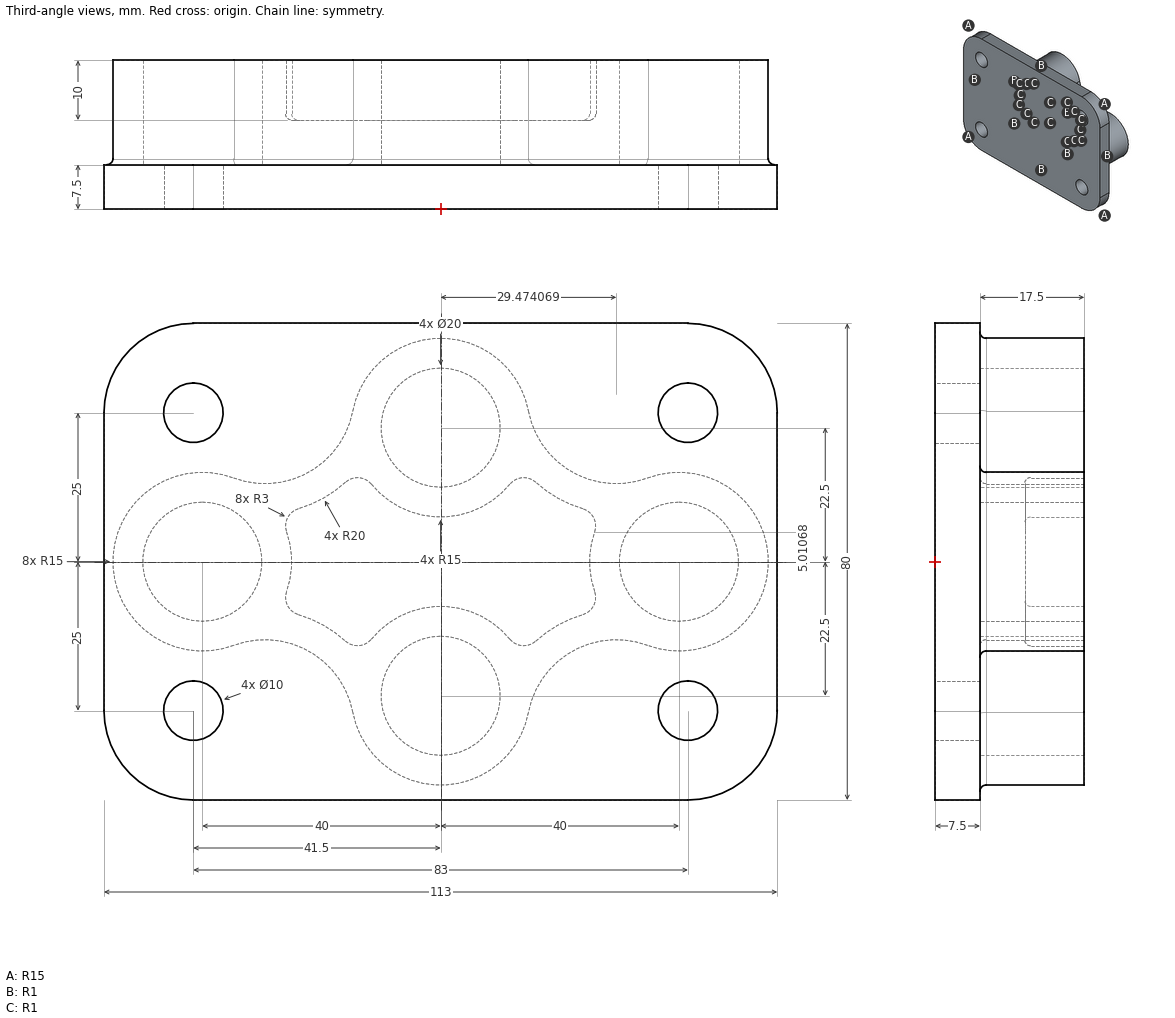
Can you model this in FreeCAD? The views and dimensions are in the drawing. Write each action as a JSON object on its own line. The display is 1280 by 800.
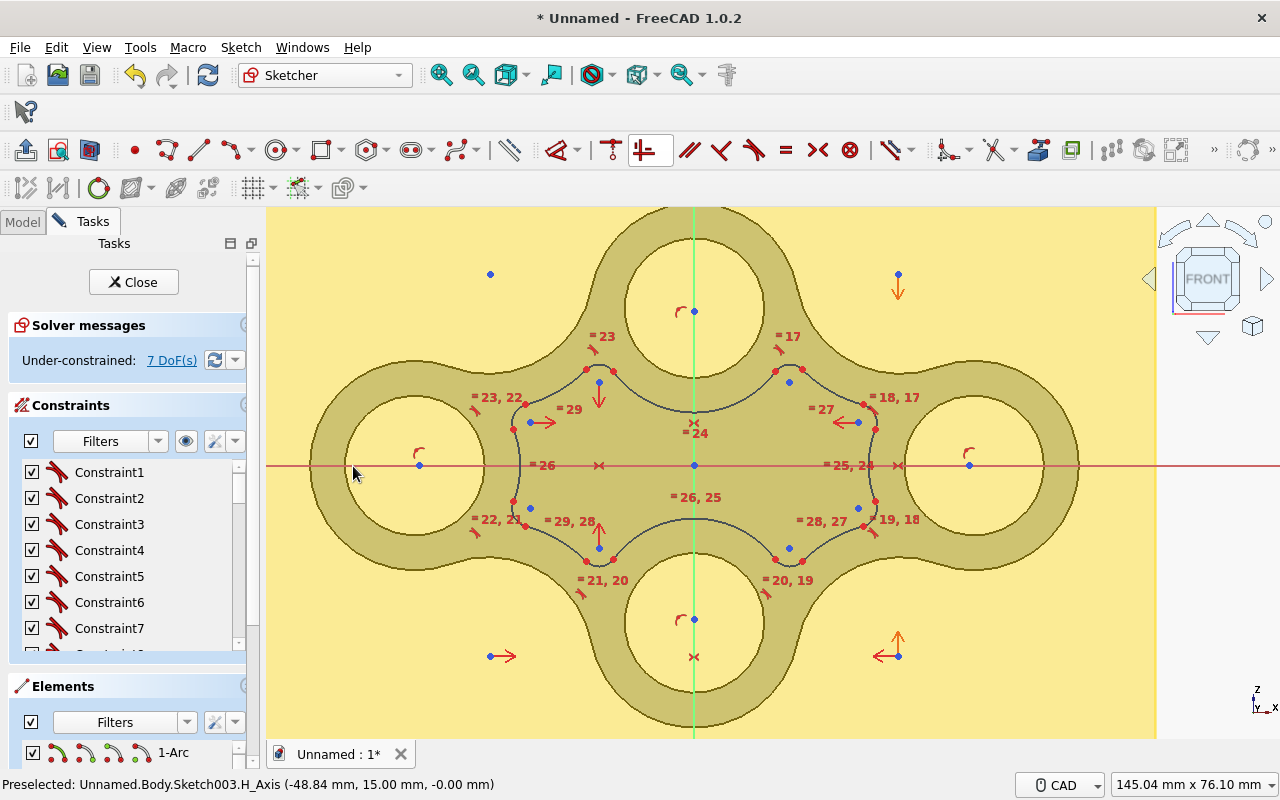
{"action": "left_click", "coordinate": [658, 406]}
{"action": "left_click", "coordinate": [646, 436]}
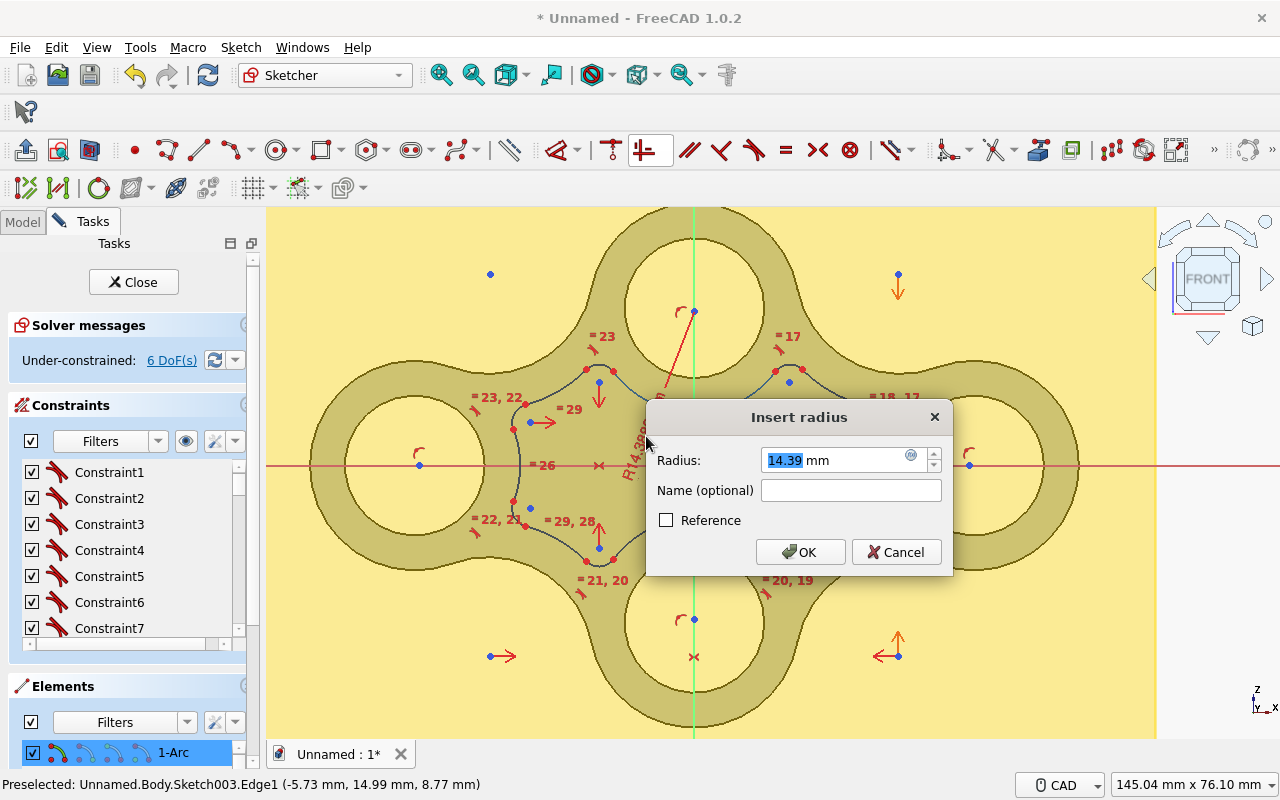
{"action": "type", "text": "15"}
{"action": "key", "text": "Return"}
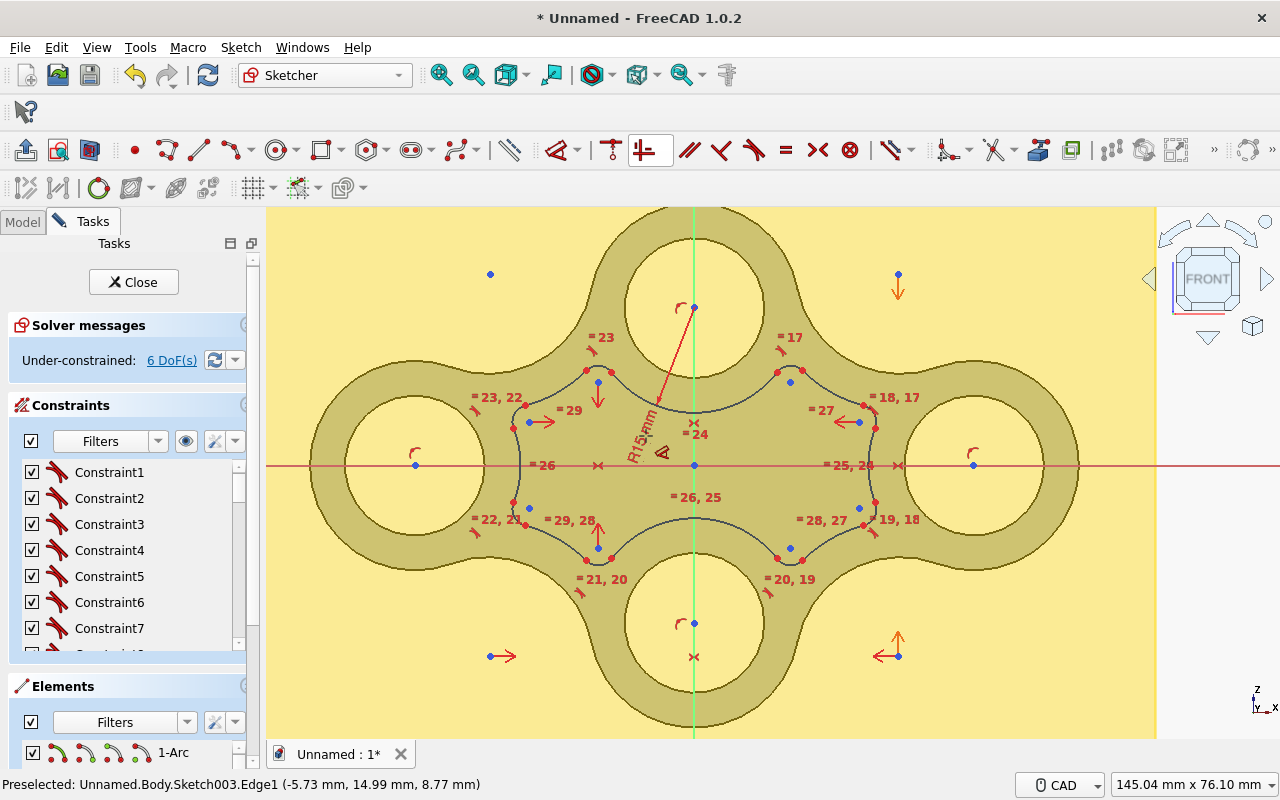
{"action": "scroll", "coordinate": [790, 366], "scroll_direction": "up", "scroll_amount": 4}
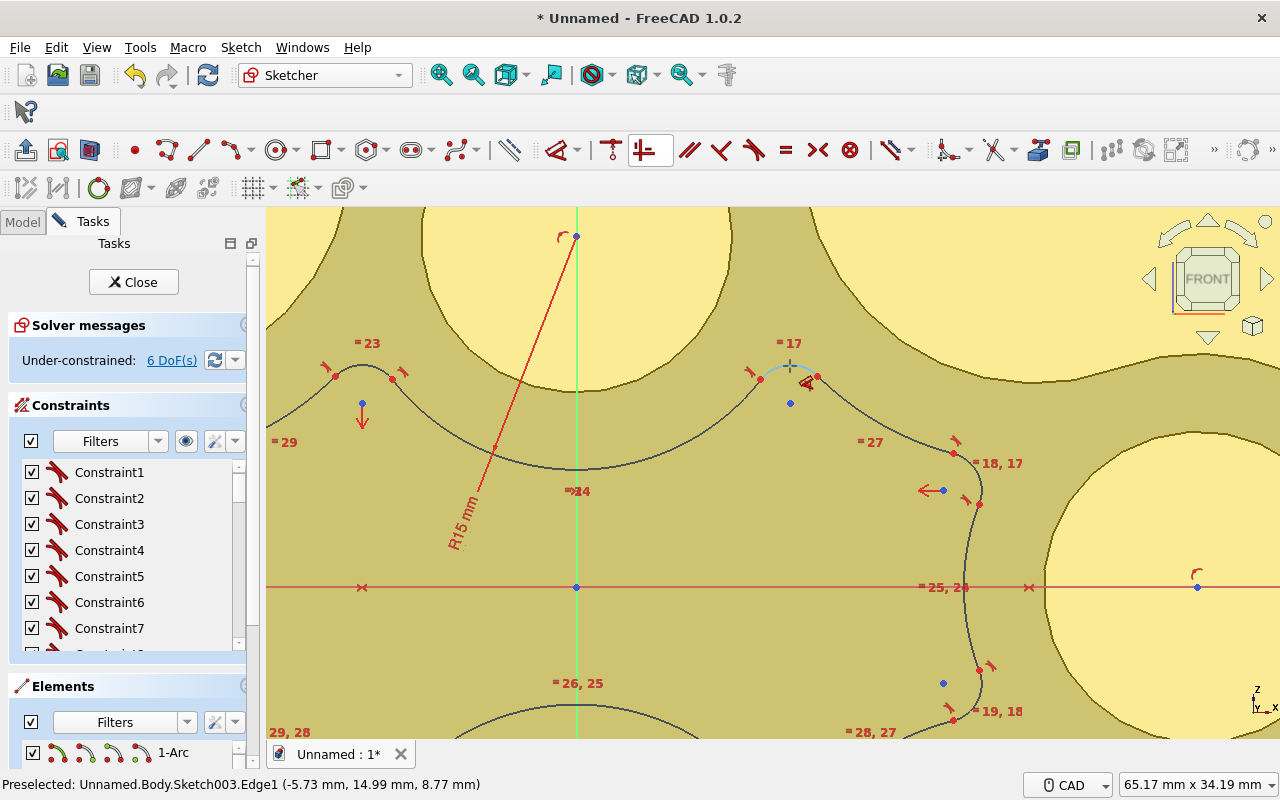
{"action": "left_click", "coordinate": [789, 365]}
{"action": "left_click", "coordinate": [787, 333]}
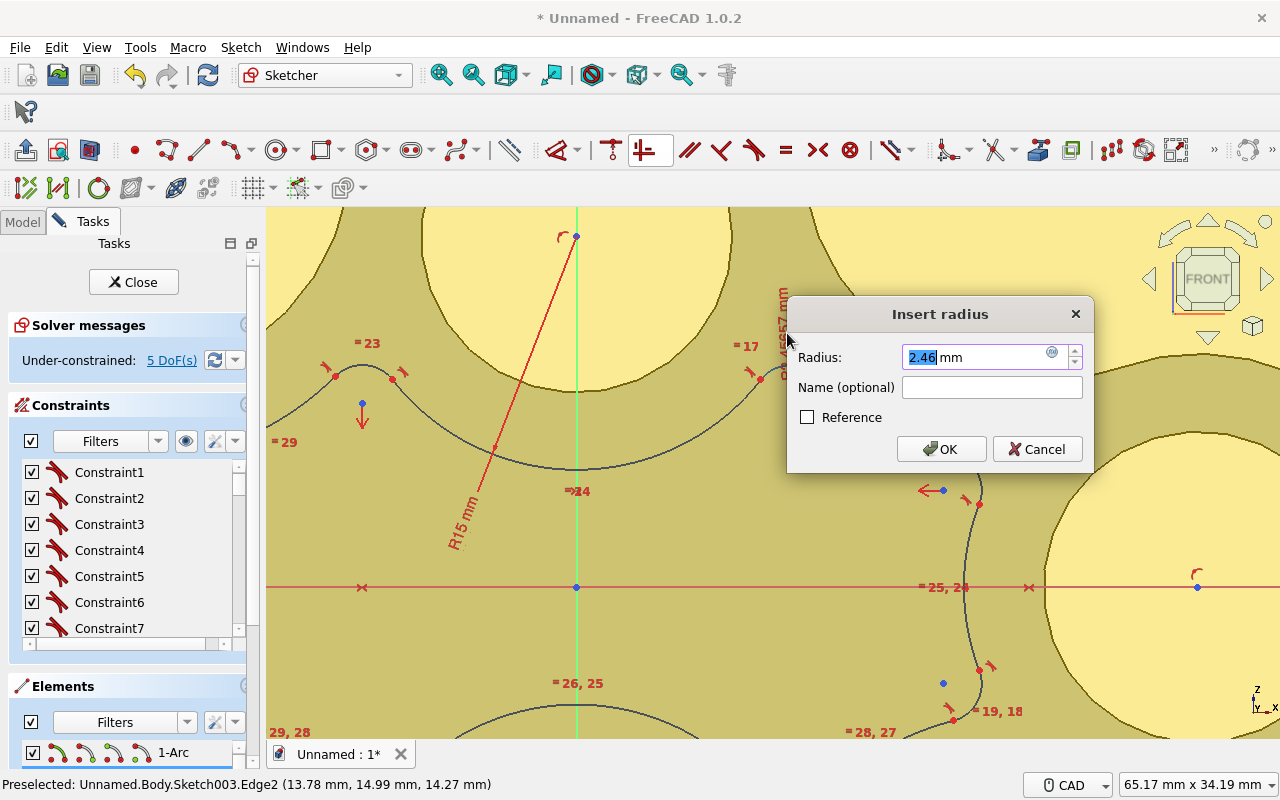
{"action": "type", "text": "3"}
{"action": "key", "text": "Return"}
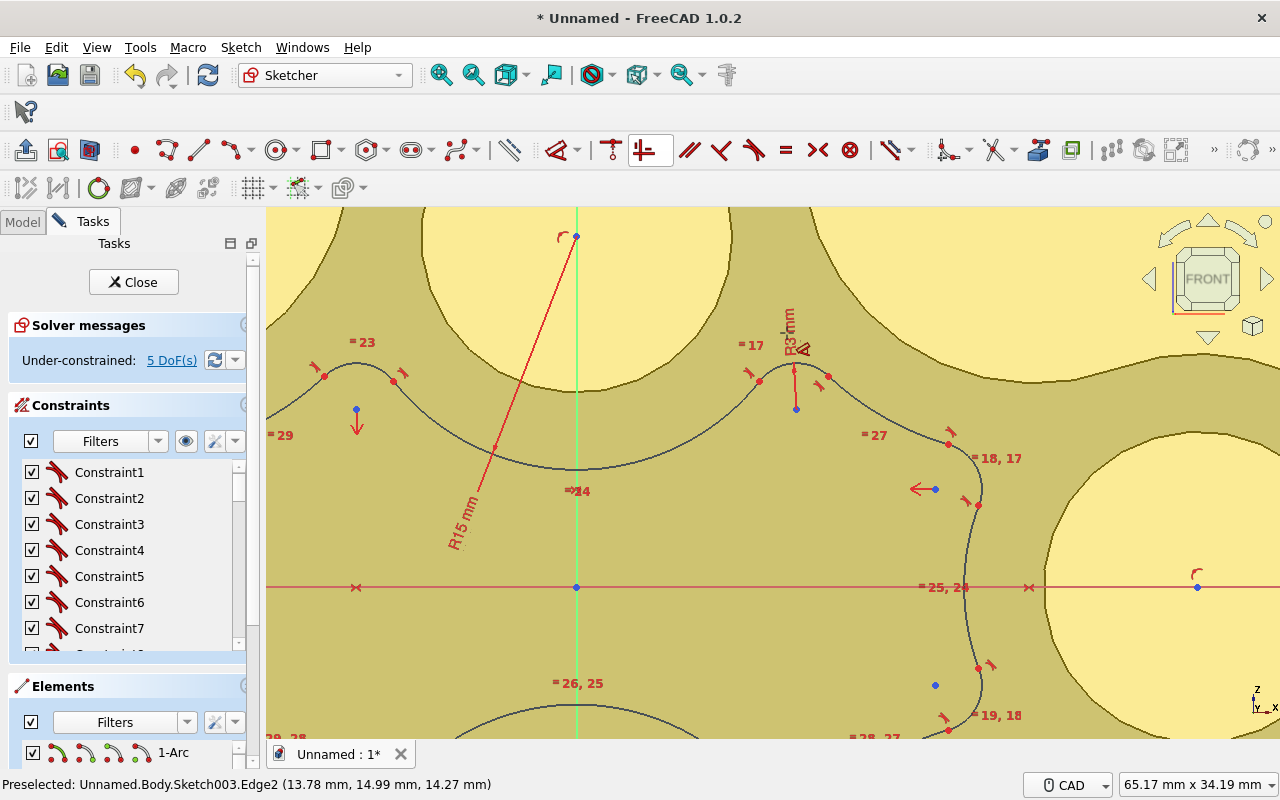
{"action": "left_click", "coordinate": [861, 402]}
{"action": "left_click", "coordinate": [843, 428]}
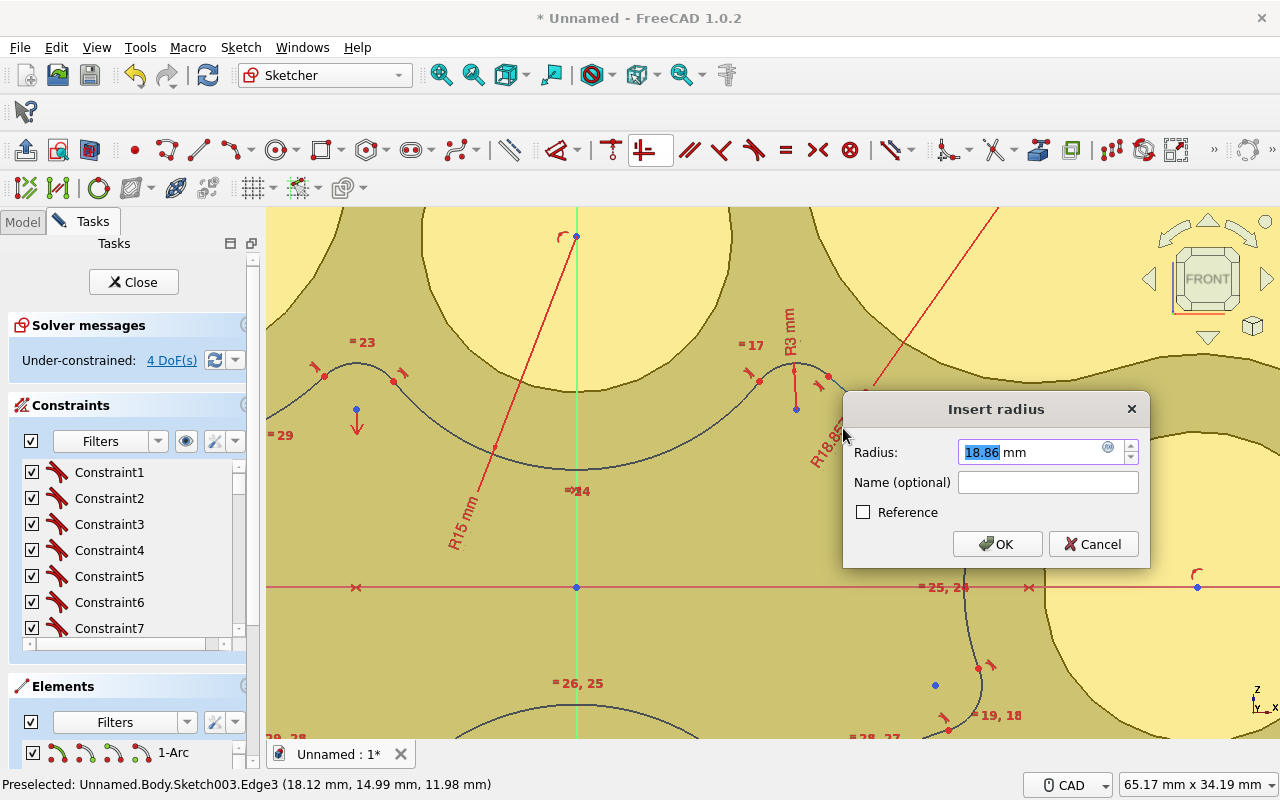
{"action": "type", "text": "20"}
{"action": "key", "text": "Return"}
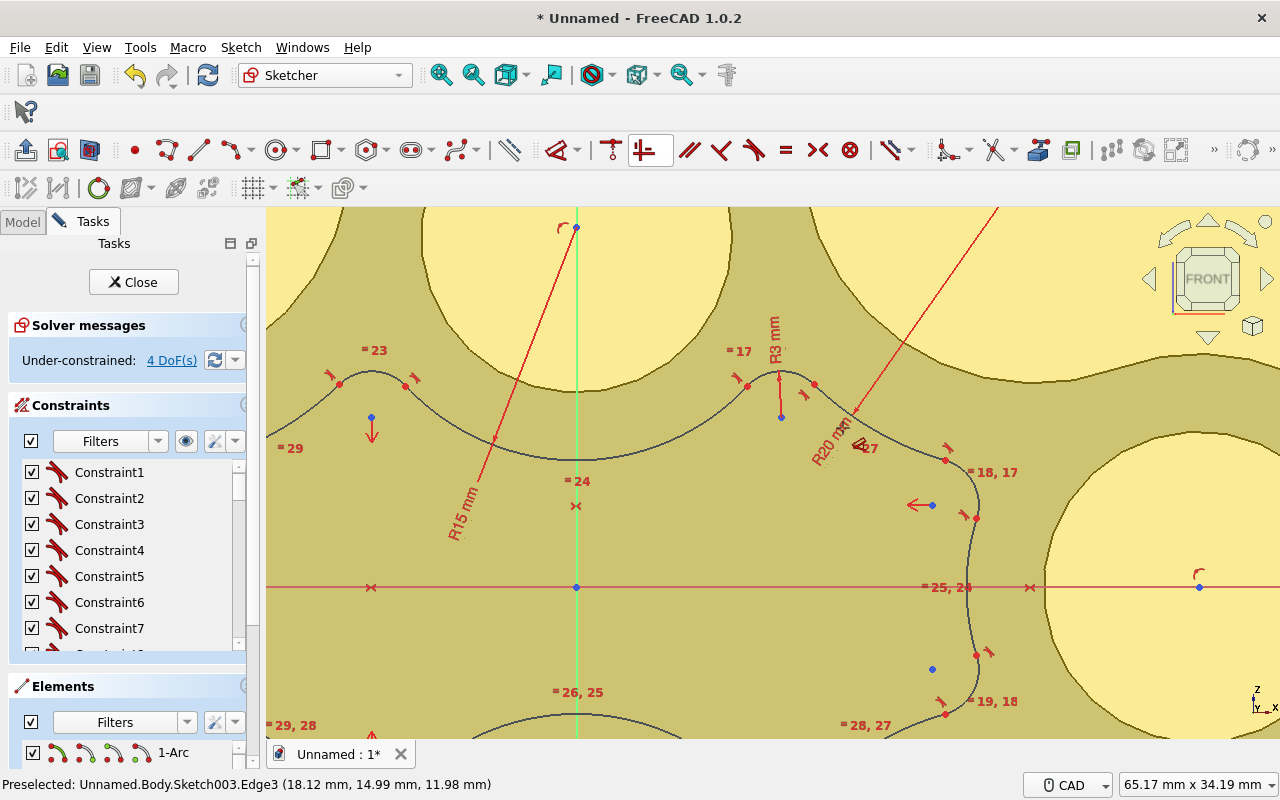
{"action": "scroll", "coordinate": [964, 241], "scroll_direction": "down", "scroll_amount": 2}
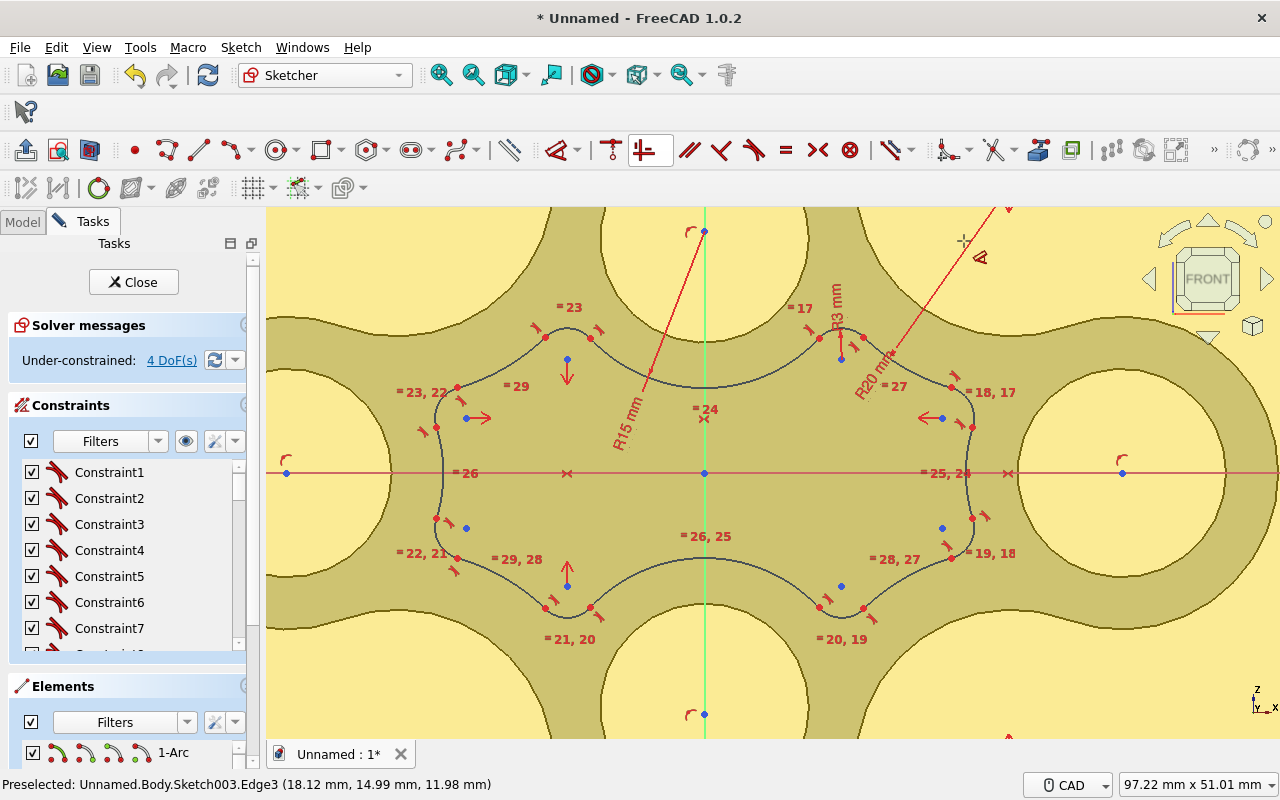
{"action": "scroll", "coordinate": [370, 473], "scroll_direction": "down", "scroll_amount": 1}